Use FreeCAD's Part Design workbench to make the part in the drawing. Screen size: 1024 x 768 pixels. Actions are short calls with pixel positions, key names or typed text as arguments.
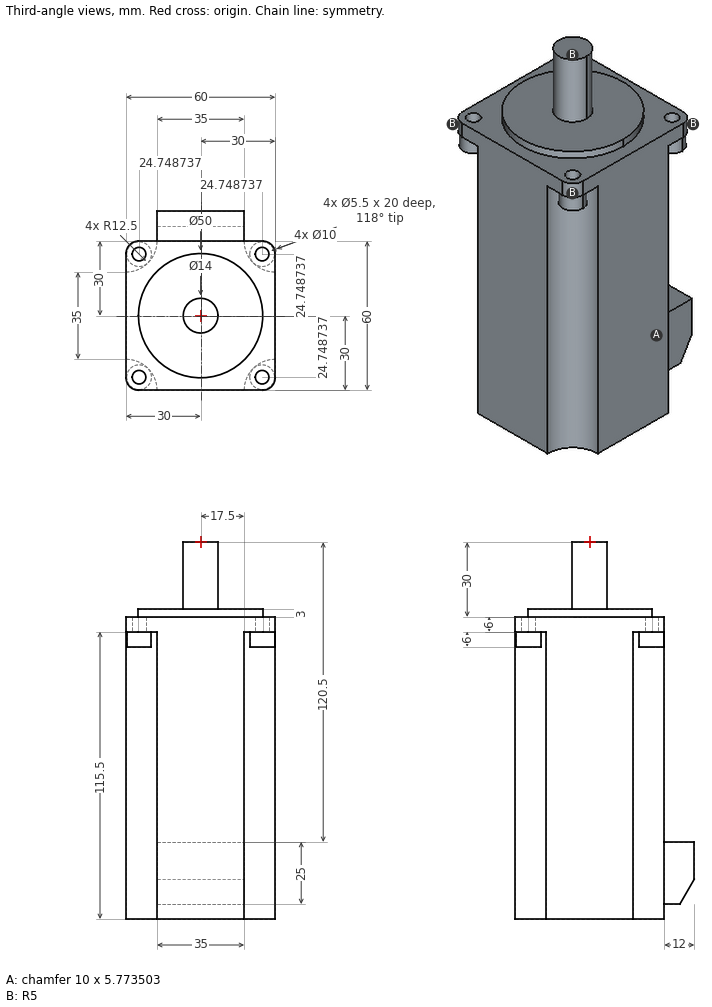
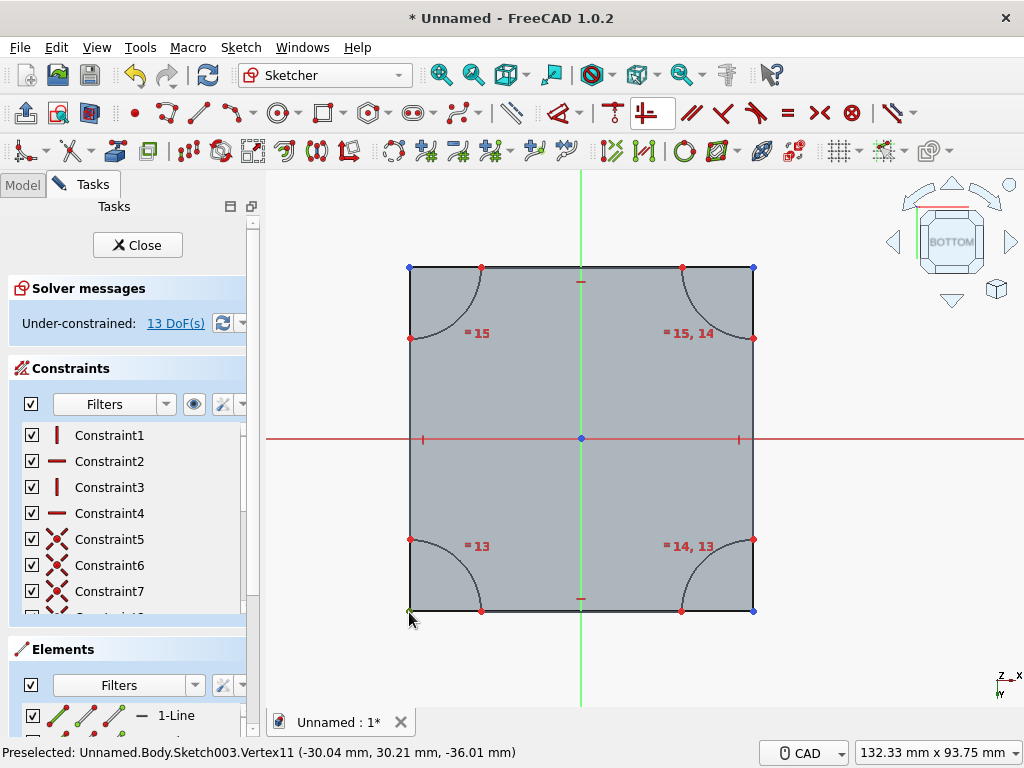
click(754, 612)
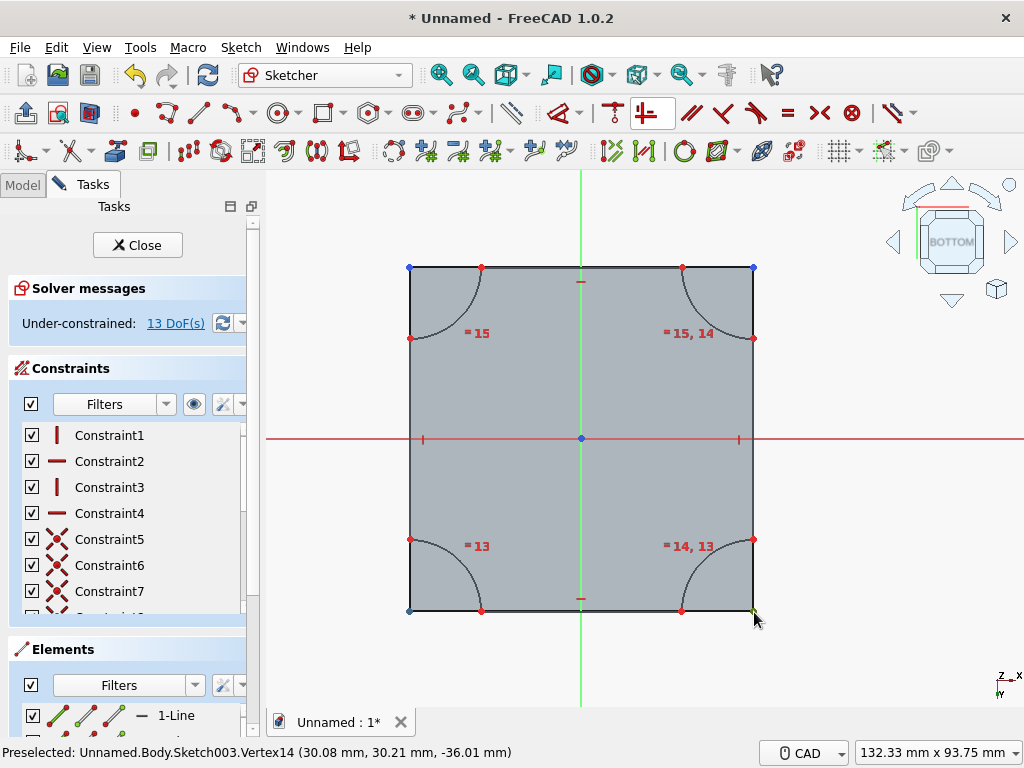
click(581, 645)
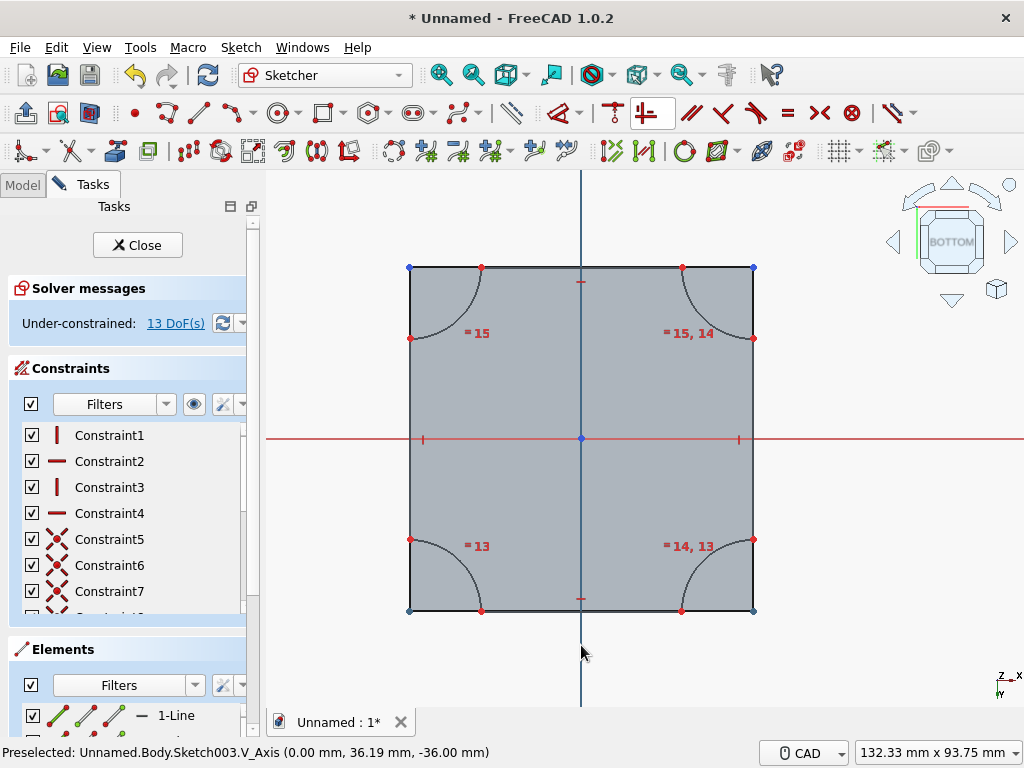
click(820, 114)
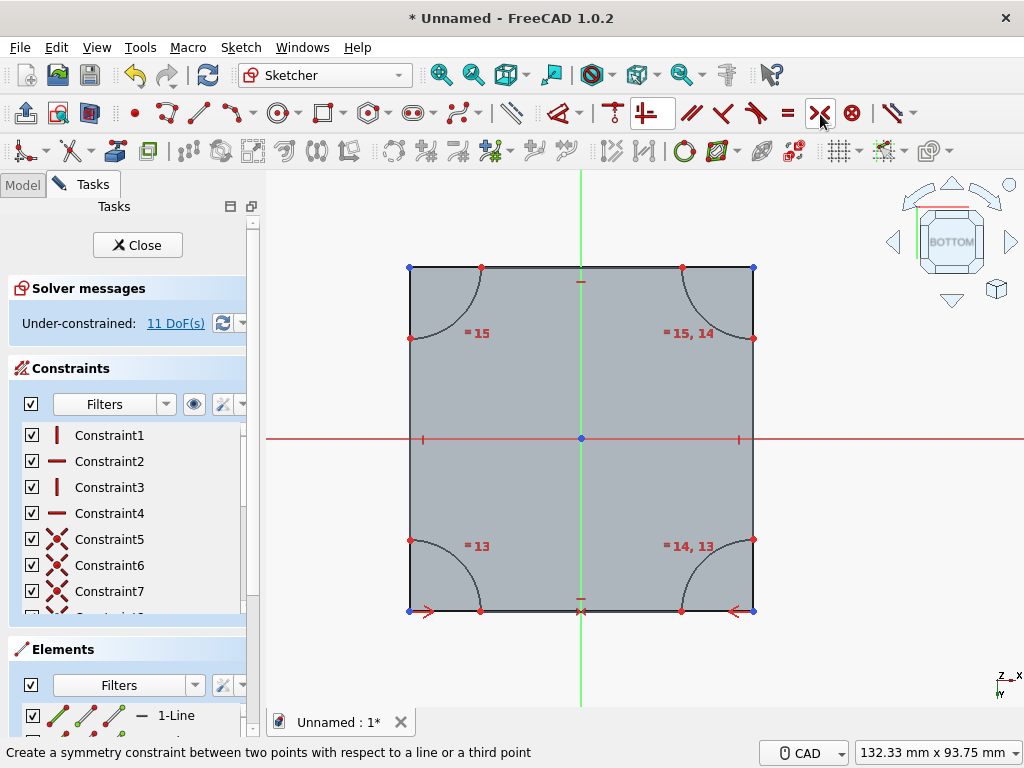
click(754, 612)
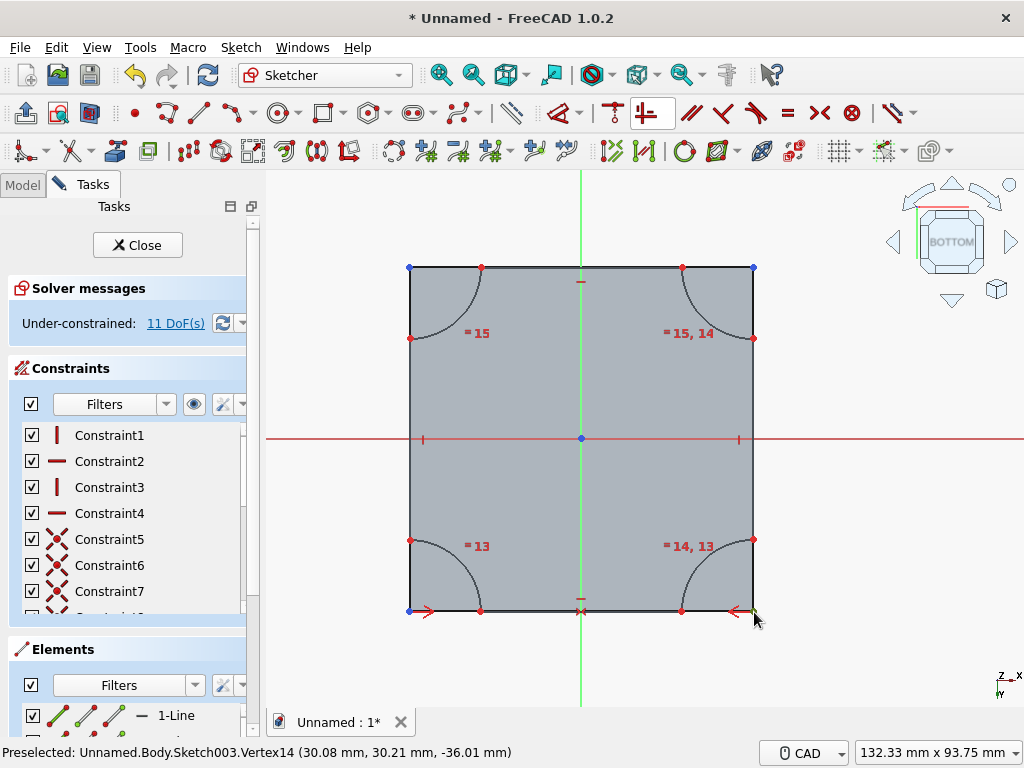
click(754, 267)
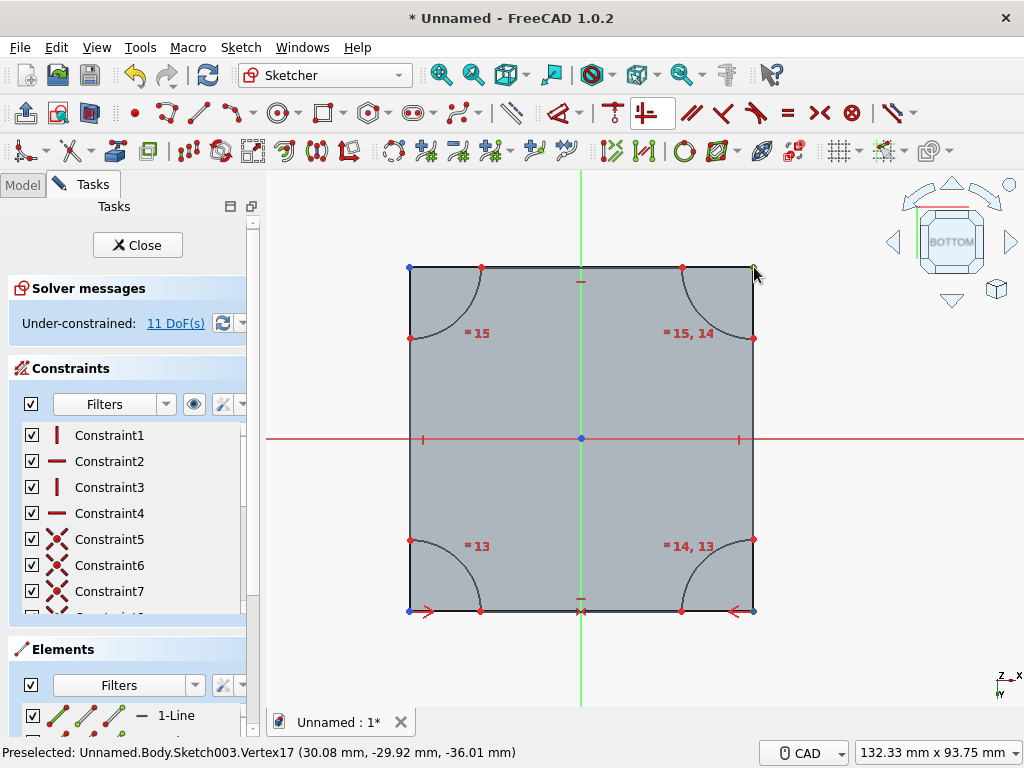
click(334, 439)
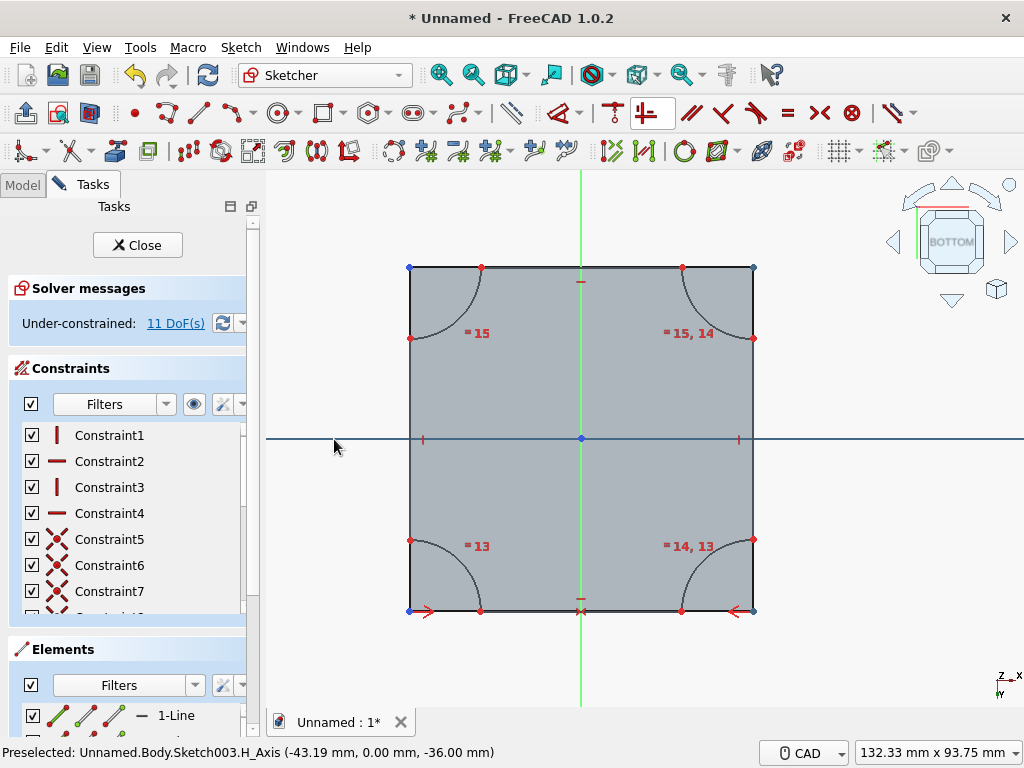
click(820, 114)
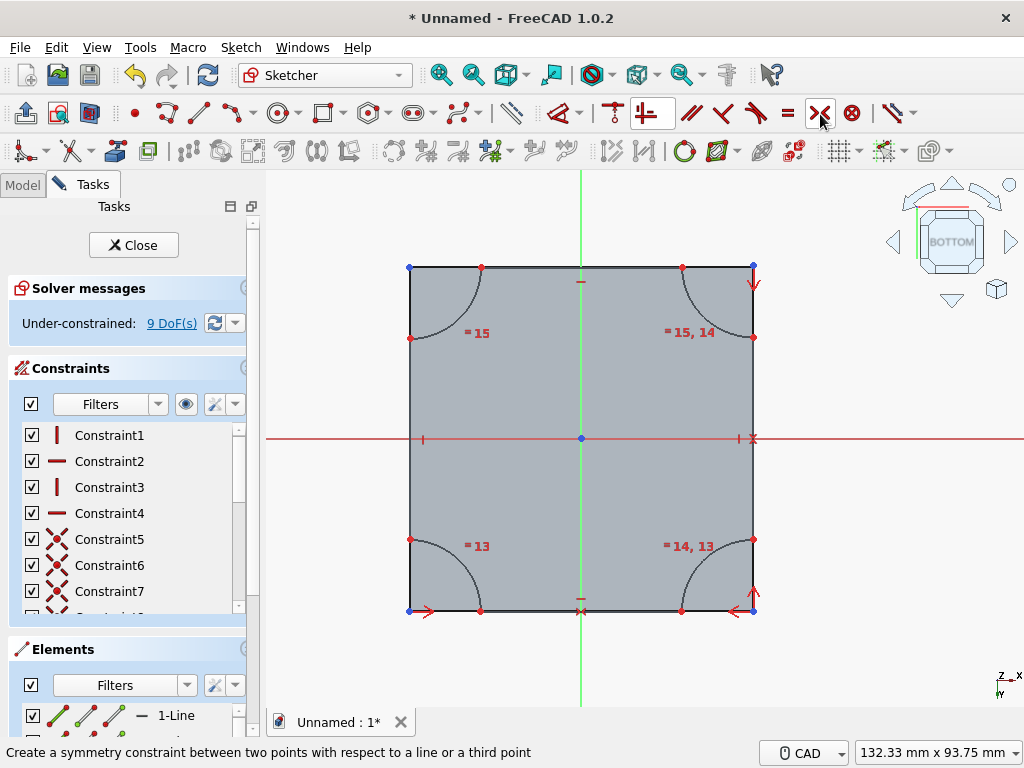
click(409, 612)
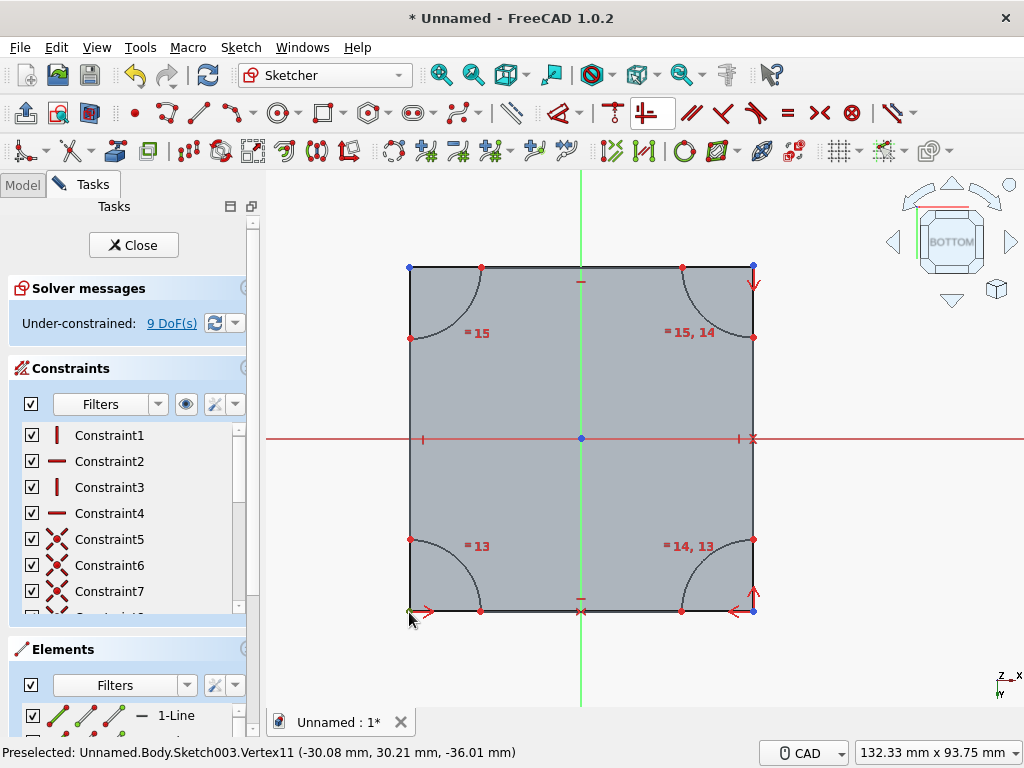
click(409, 267)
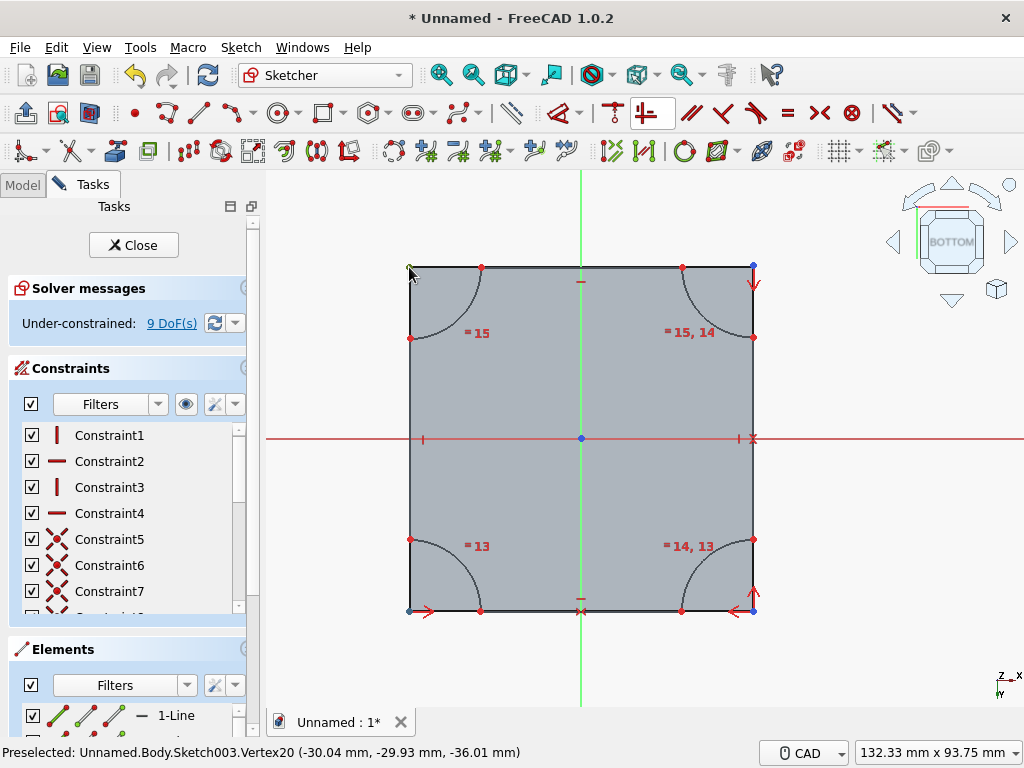
click(334, 439)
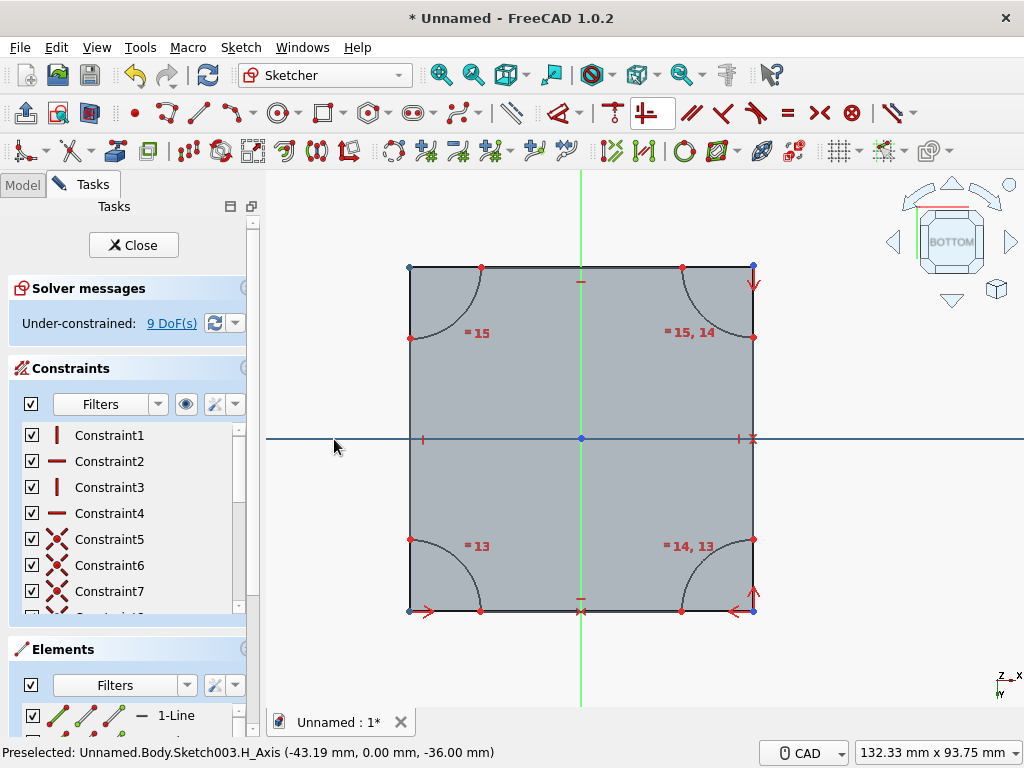
click(820, 114)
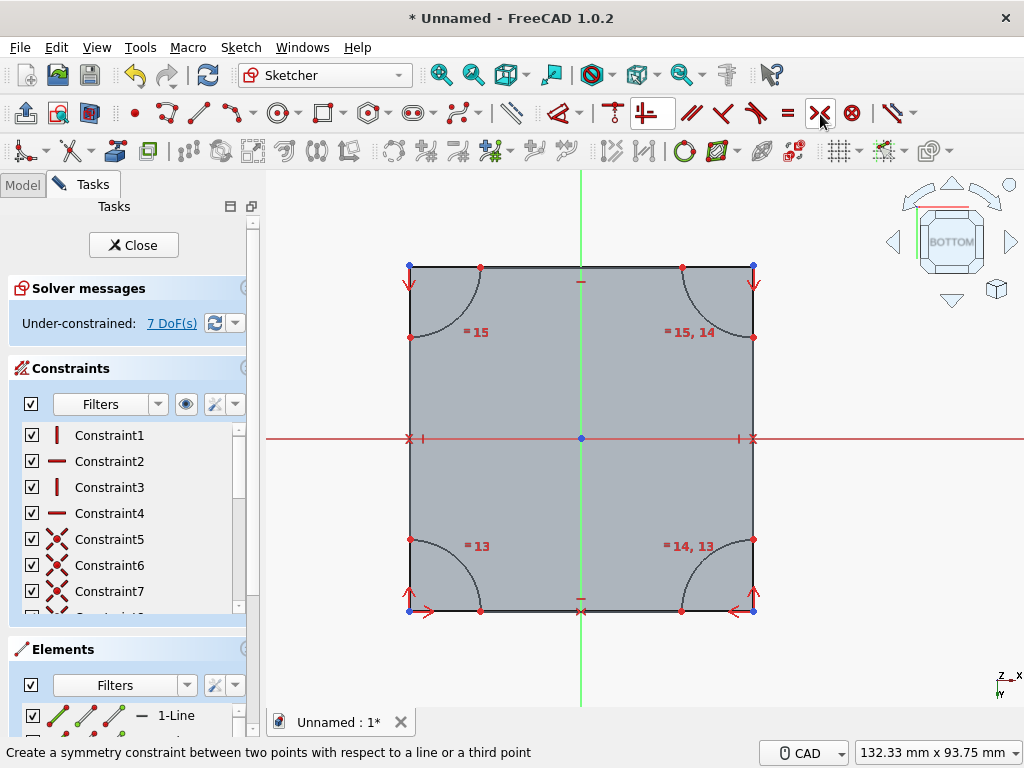
click(558, 114)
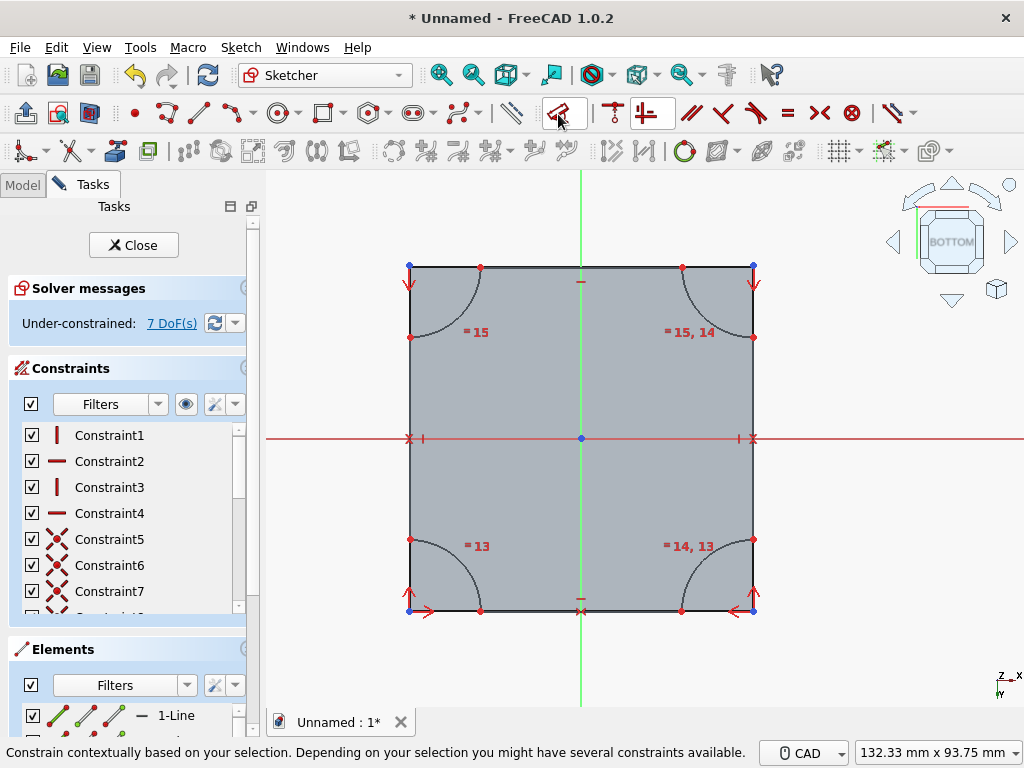
click(473, 580)
click(502, 566)